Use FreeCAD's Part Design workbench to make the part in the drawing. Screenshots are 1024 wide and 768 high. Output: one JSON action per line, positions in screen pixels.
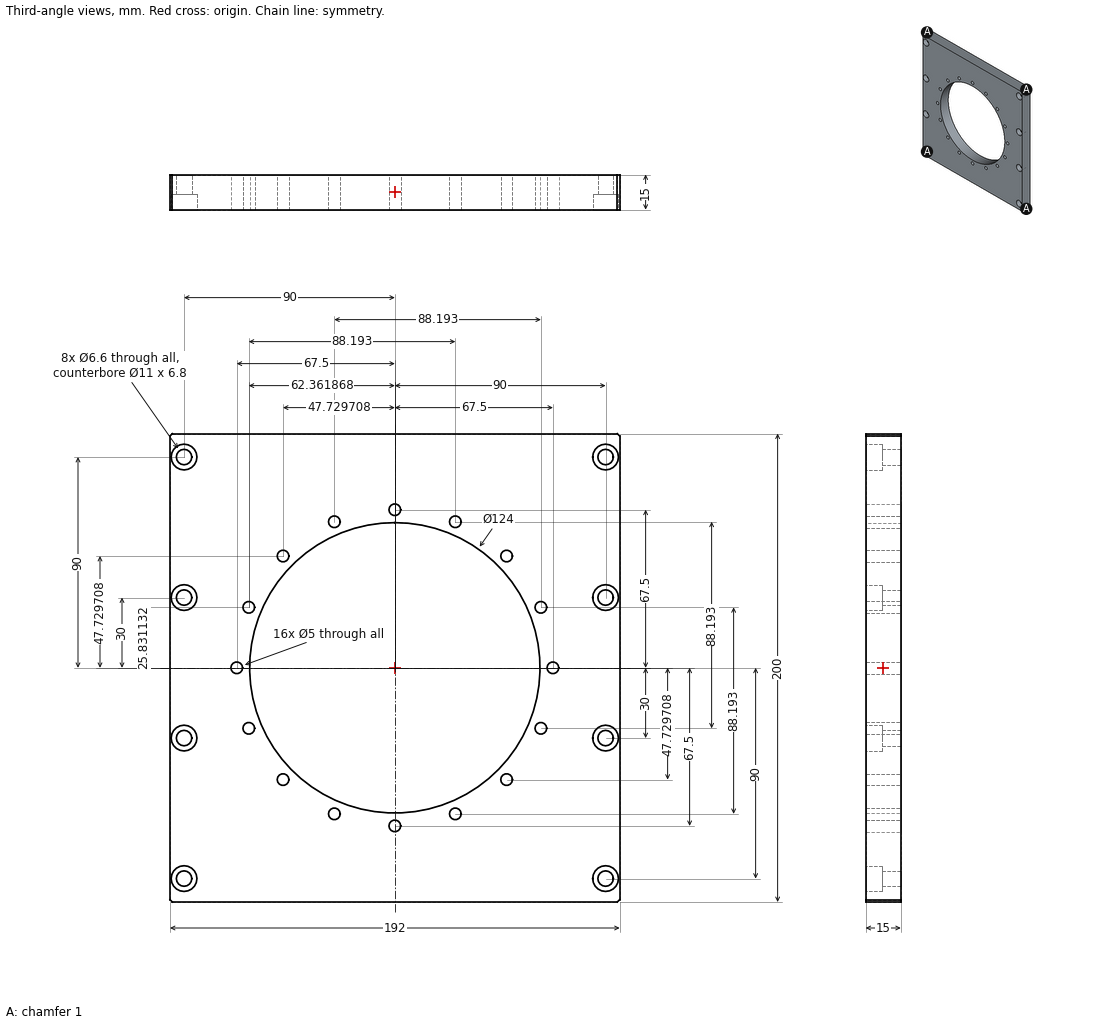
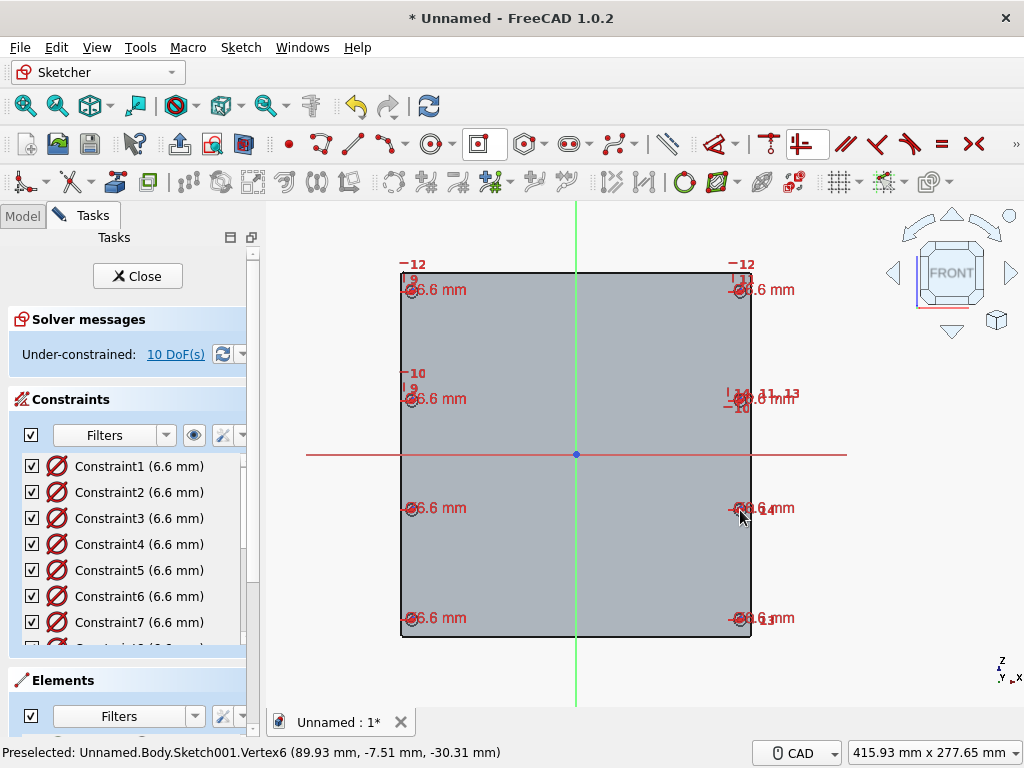
{"action": "left_click", "coordinate": [412, 401]}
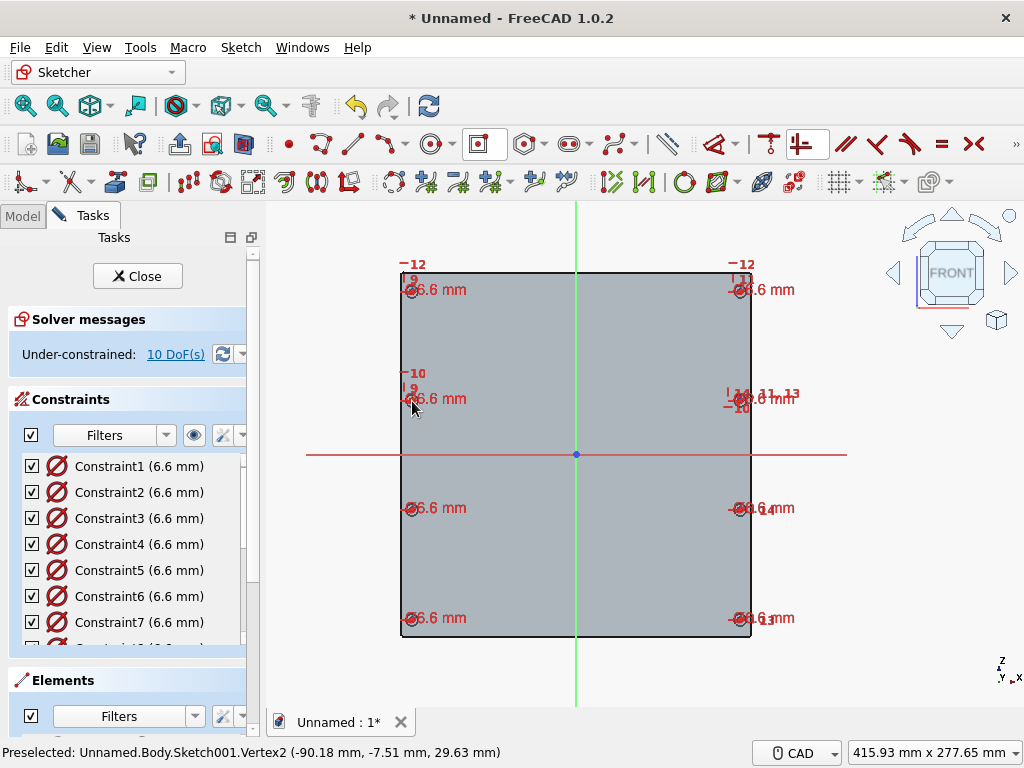
{"action": "left_click", "coordinate": [412, 510]}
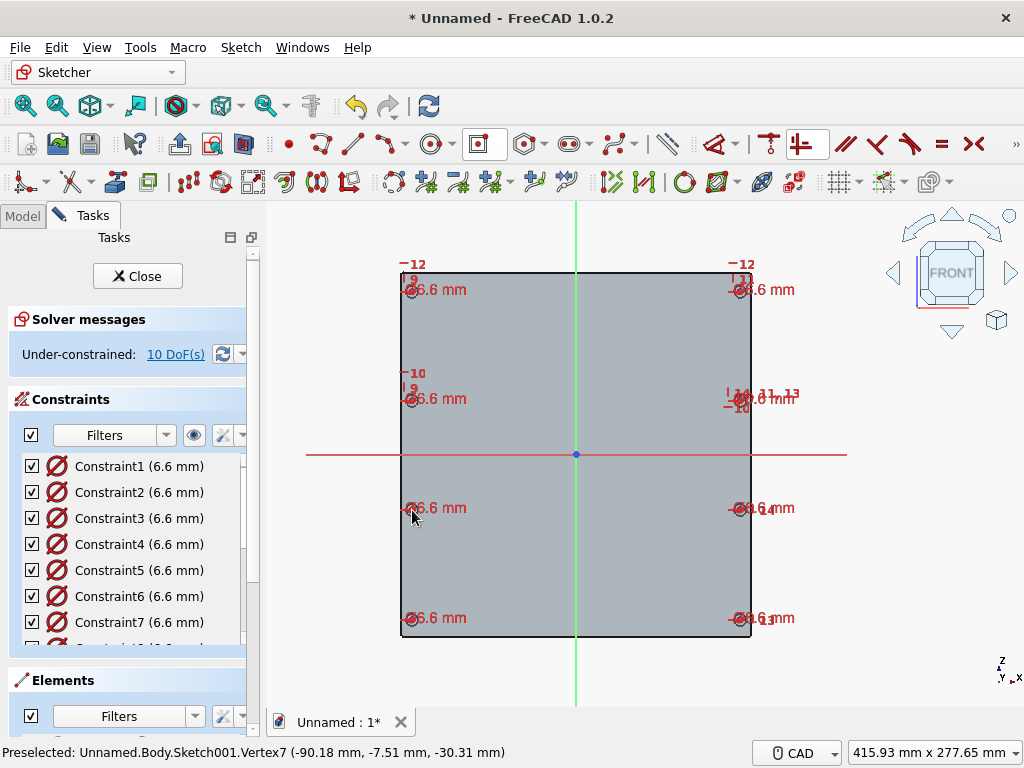
{"action": "left_click", "coordinate": [824, 144]}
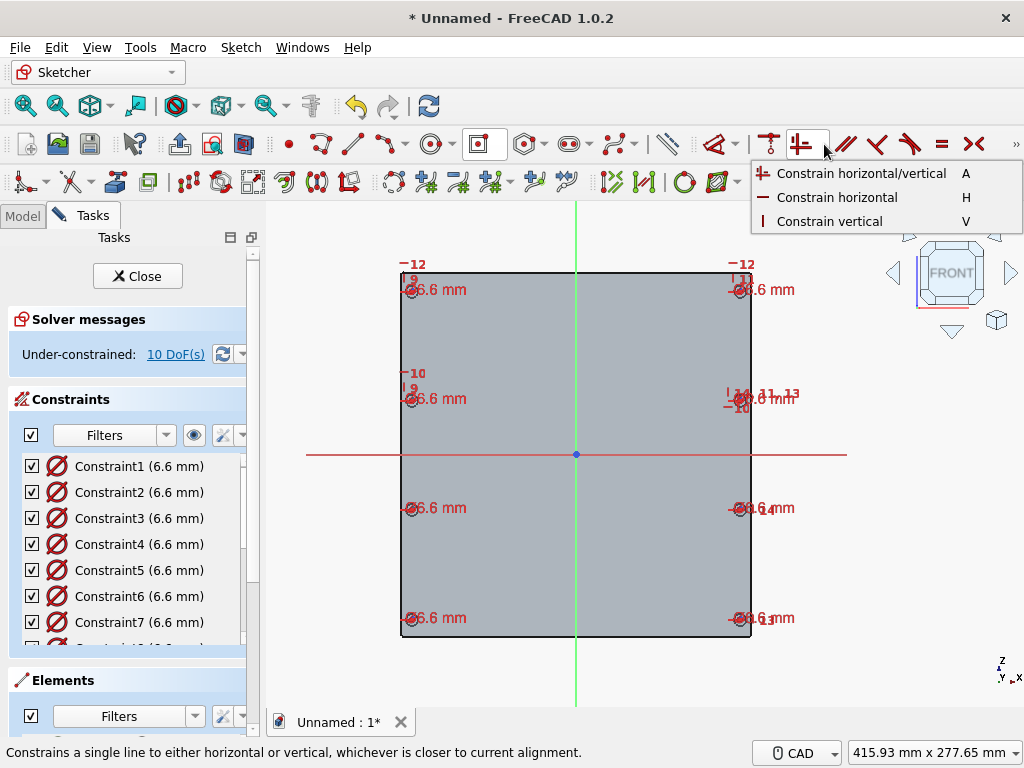
{"action": "left_click", "coordinate": [887, 221]}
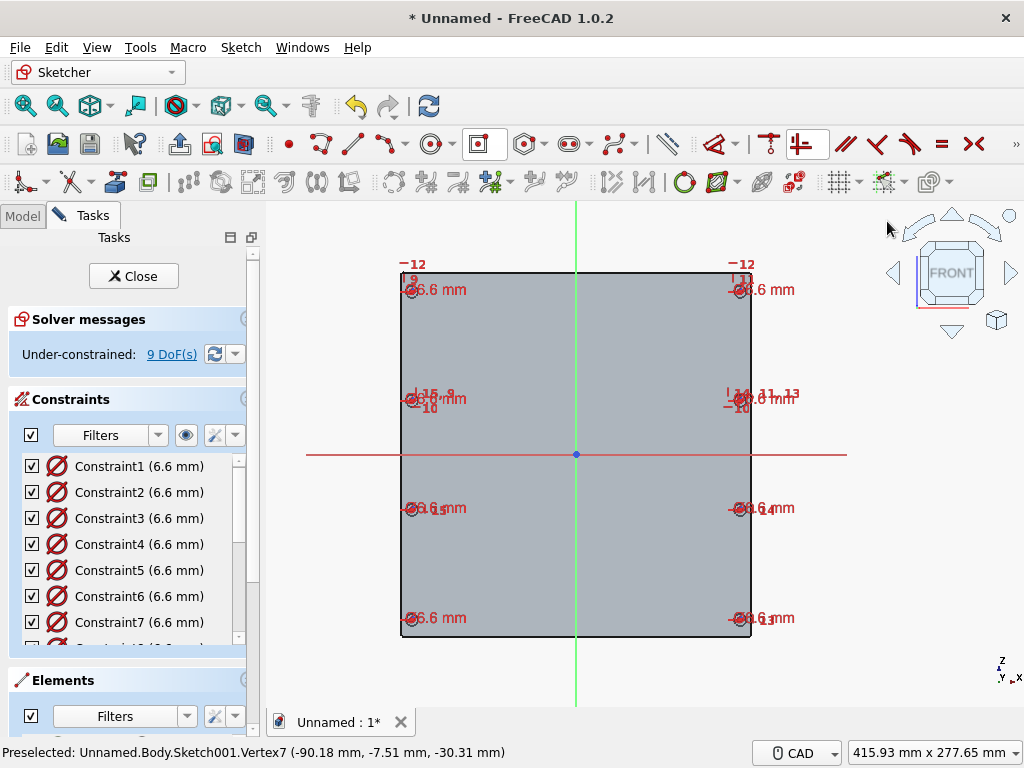
{"action": "left_click", "coordinate": [740, 510]}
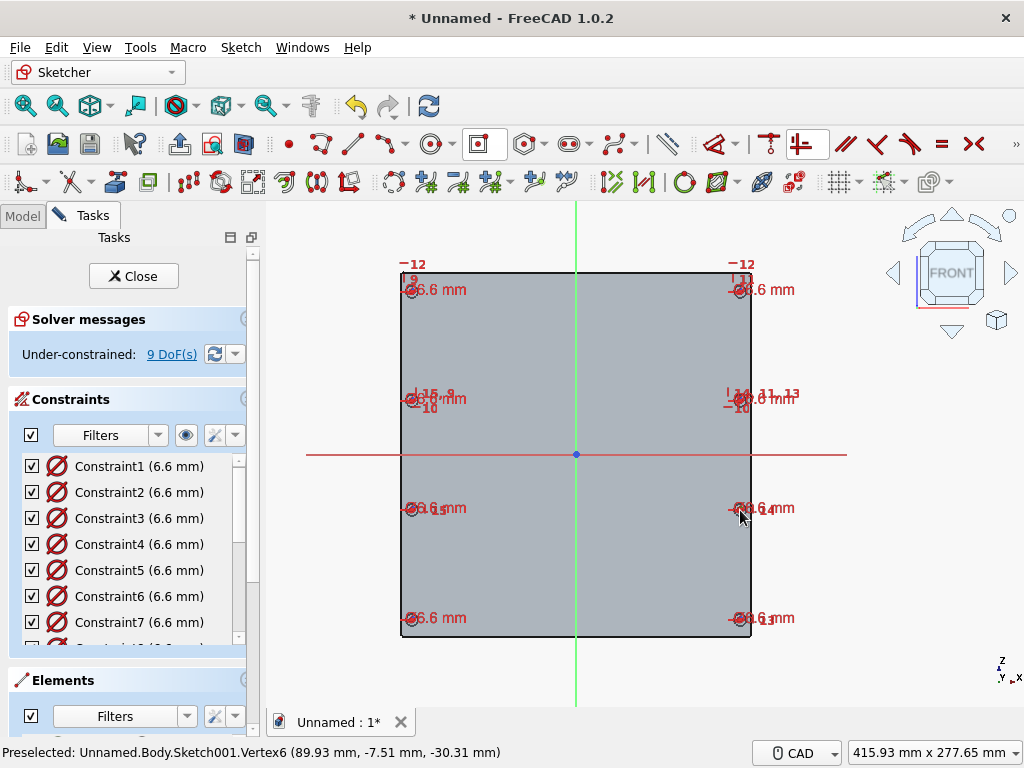
{"action": "left_click", "coordinate": [412, 510]}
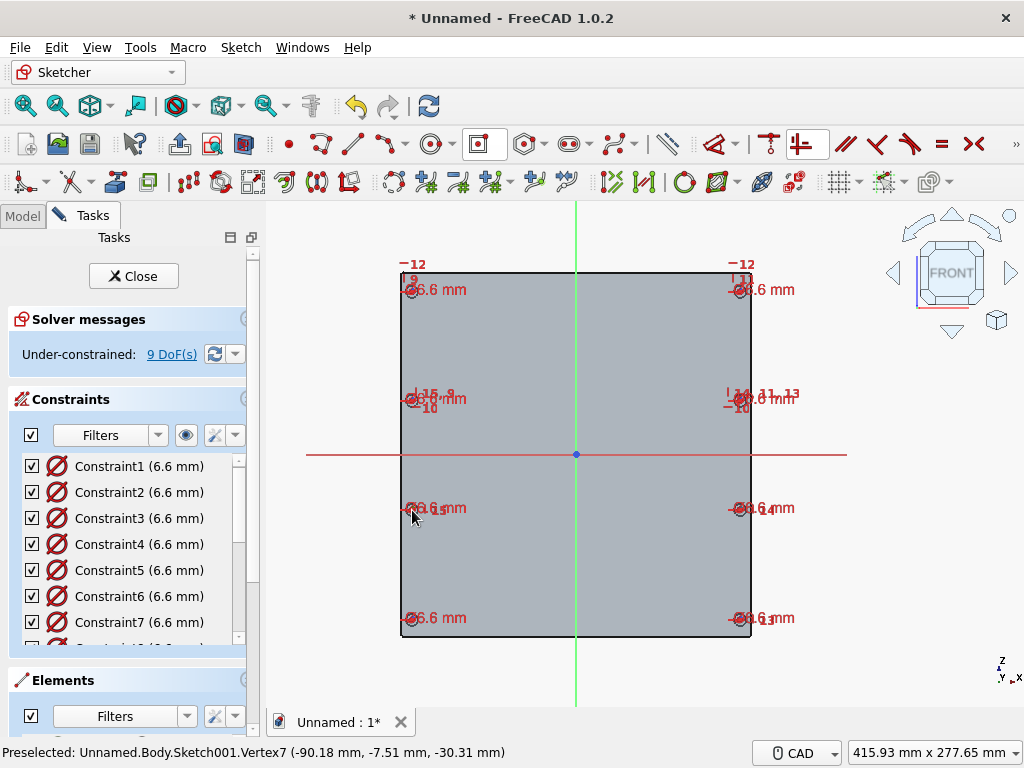
{"action": "left_click", "coordinate": [824, 144]}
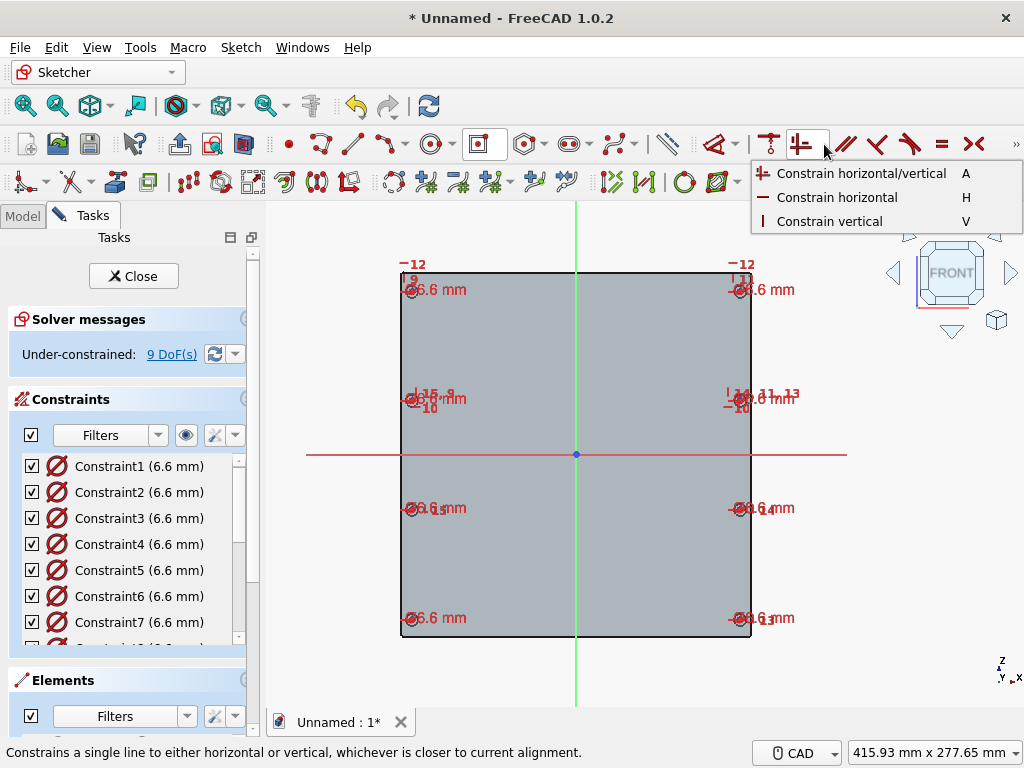
{"action": "left_click", "coordinate": [887, 197]}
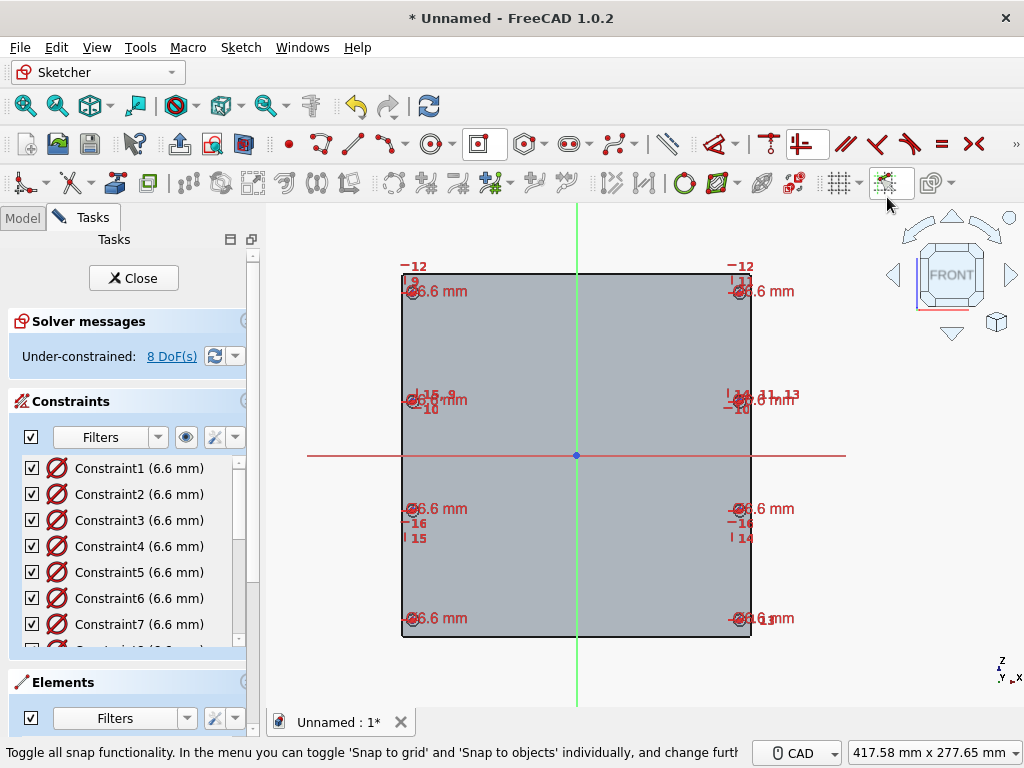
{"action": "left_click", "coordinate": [413, 511]}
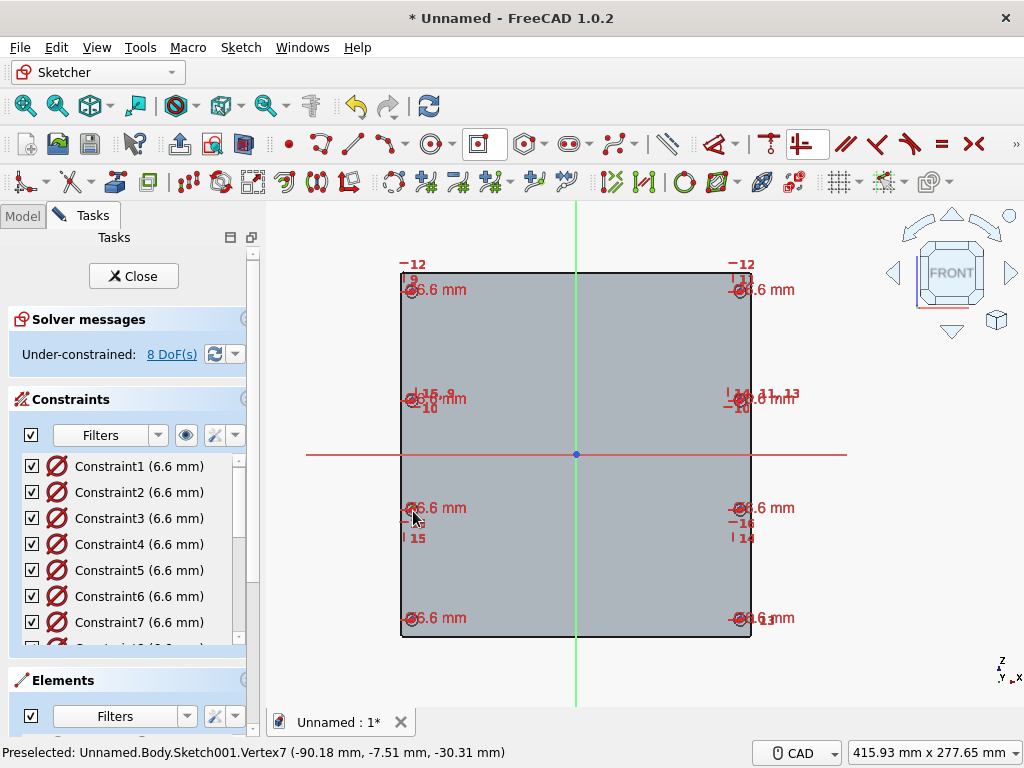
{"action": "left_click", "coordinate": [412, 620]}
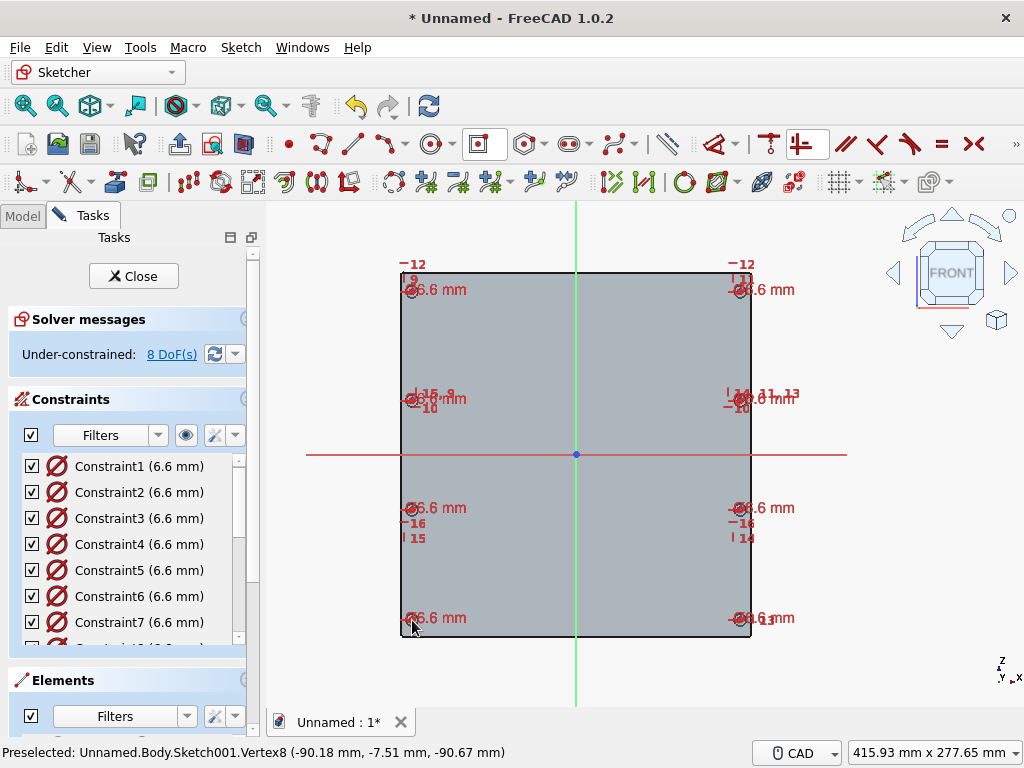
{"action": "left_click", "coordinate": [824, 144]}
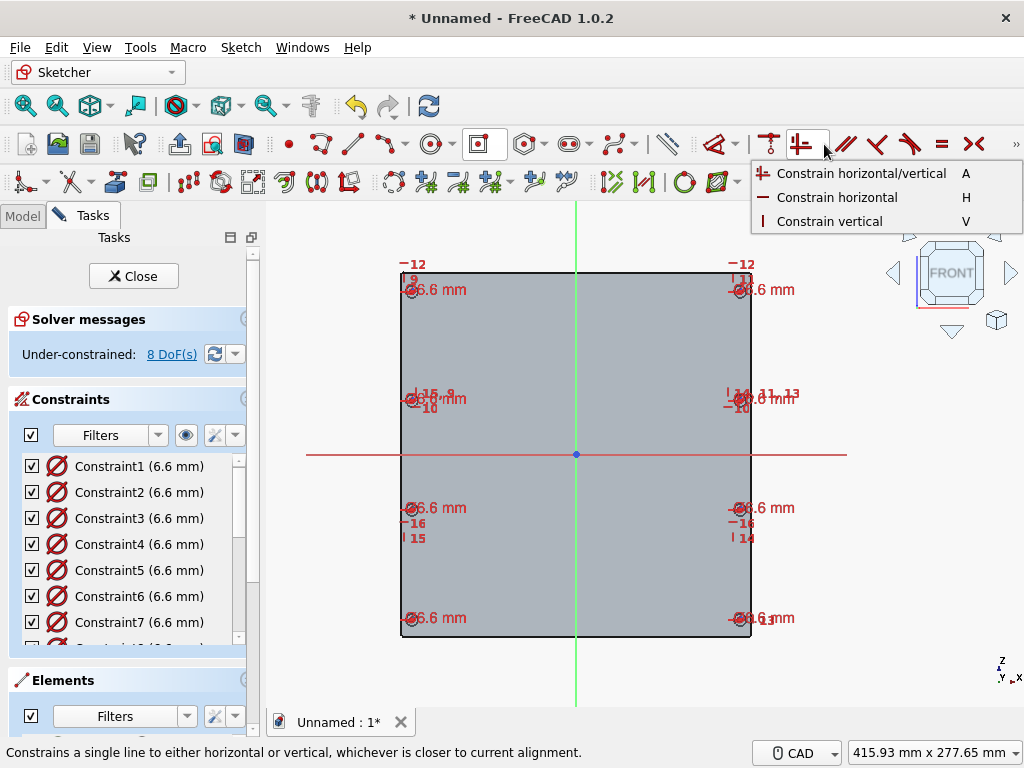
{"action": "left_click", "coordinate": [887, 221]}